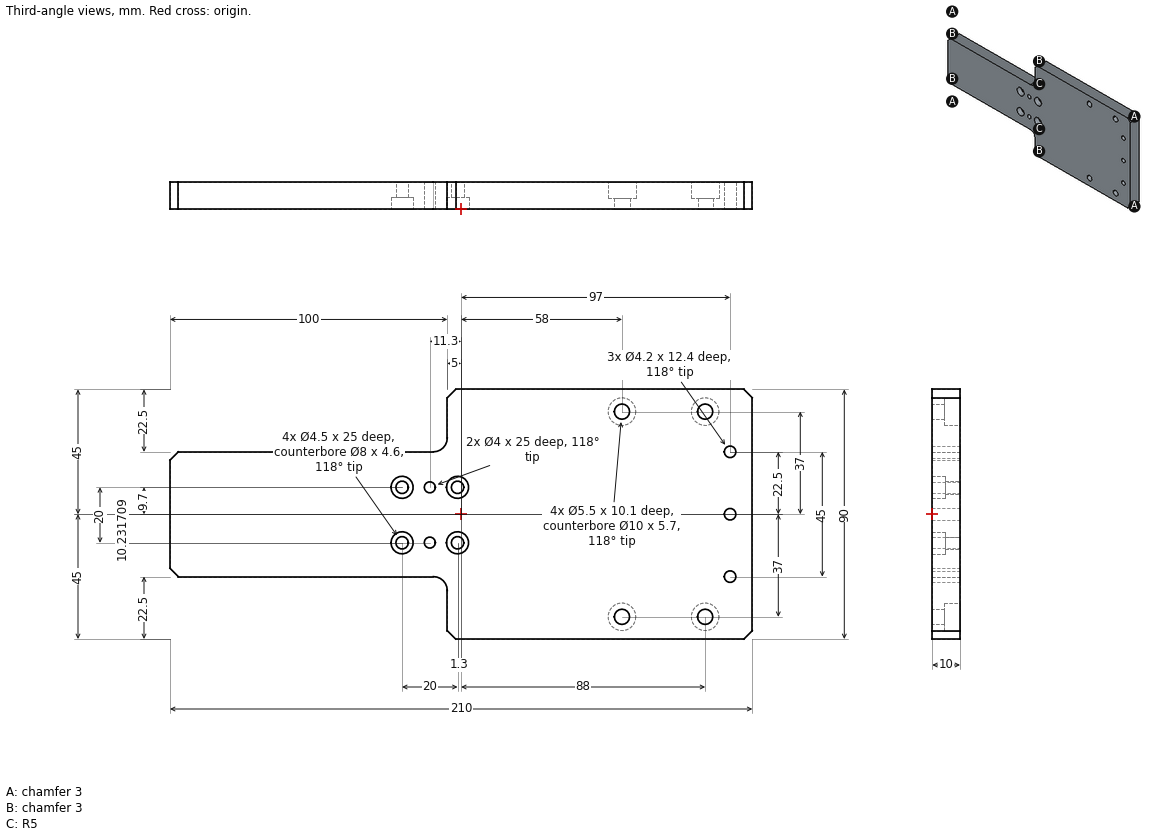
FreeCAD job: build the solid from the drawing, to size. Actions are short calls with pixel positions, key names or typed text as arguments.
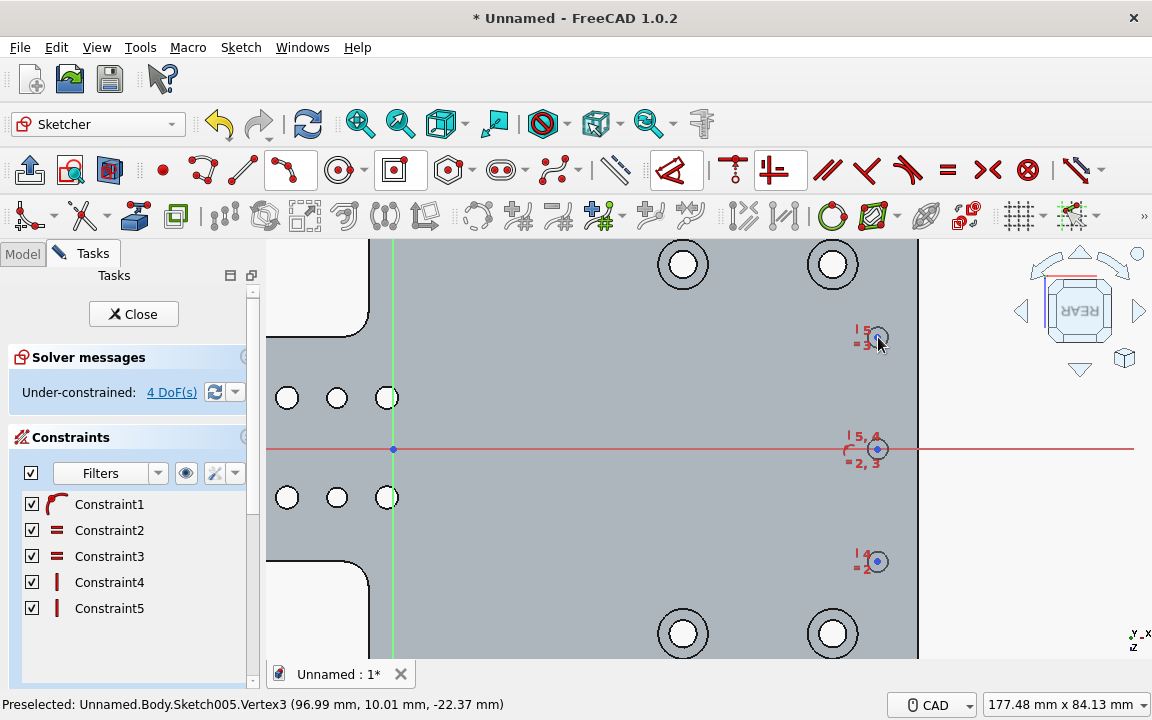
scroll(885, 555, up, 4)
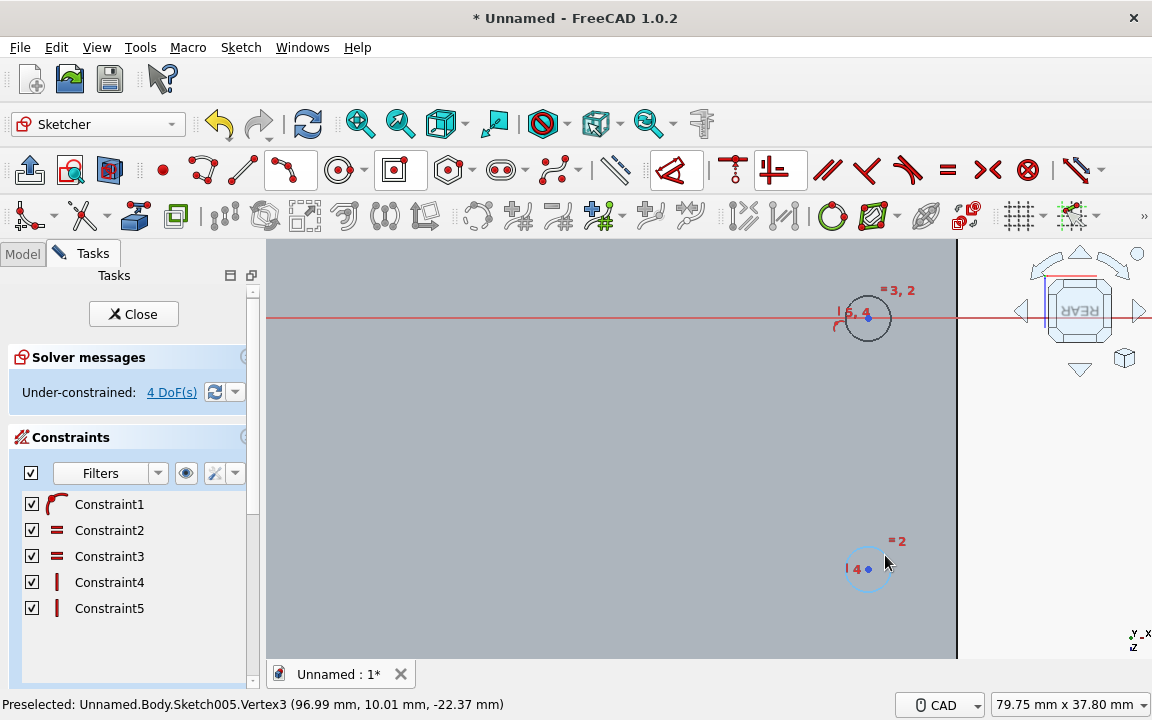
click(884, 553)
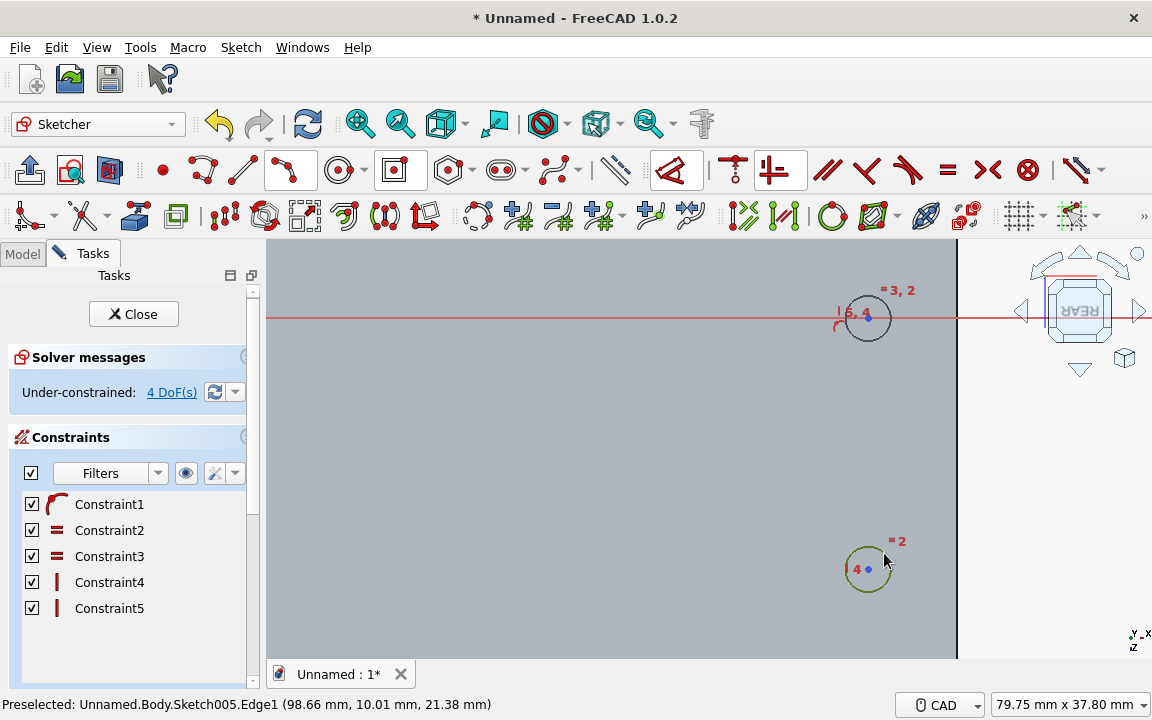
key(k)
key(o)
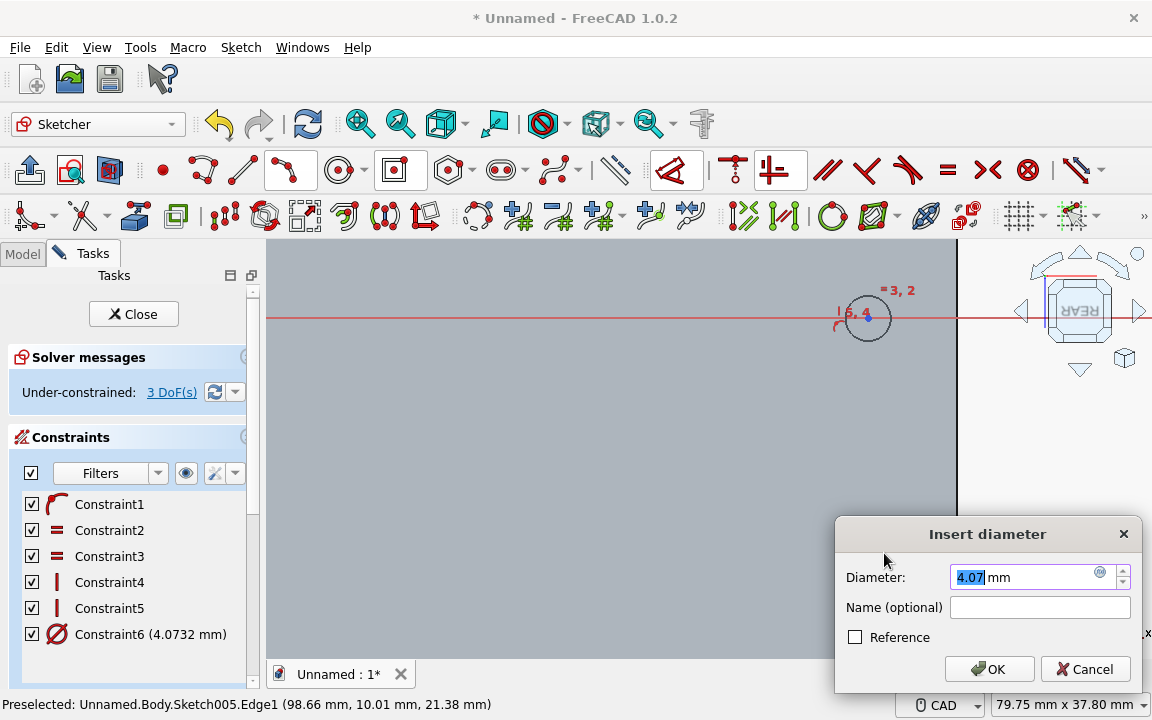
text(4.2)
key(Return)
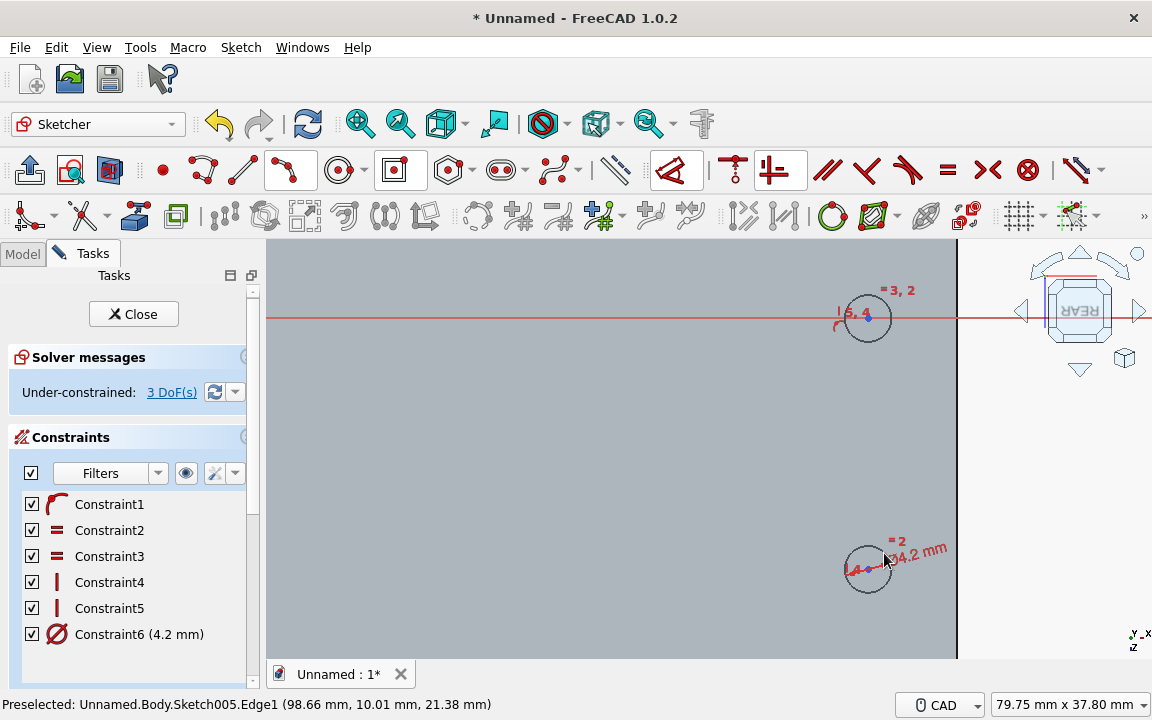
click(868, 569)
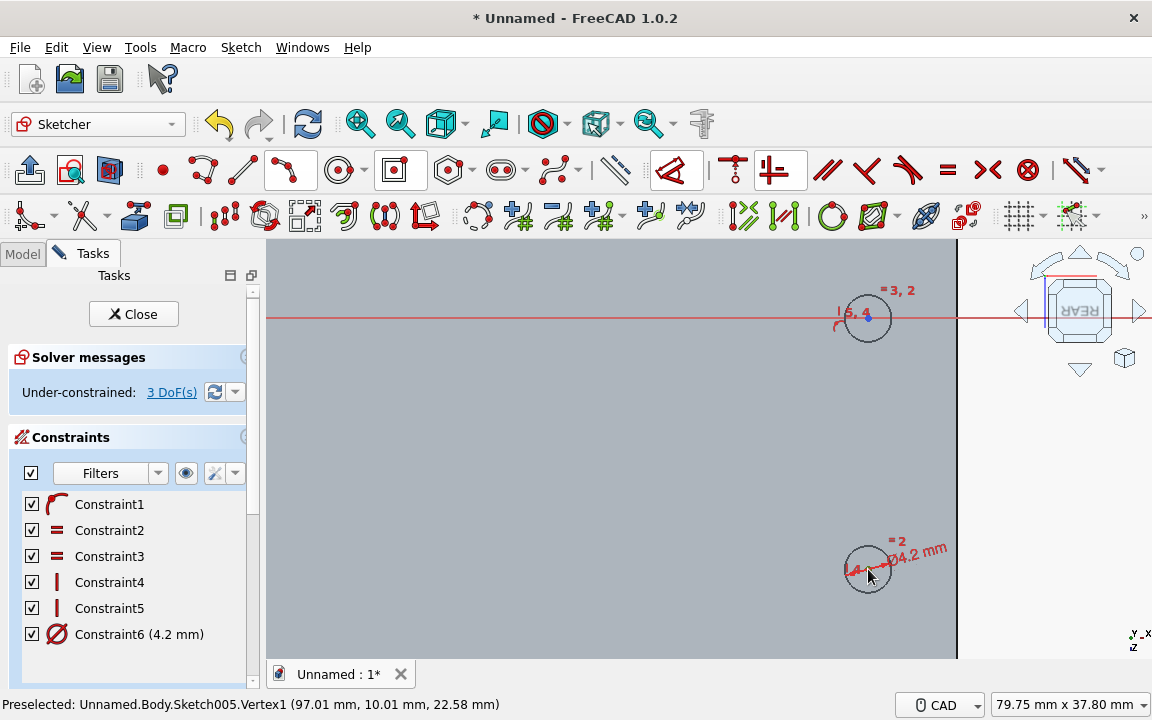
key(l)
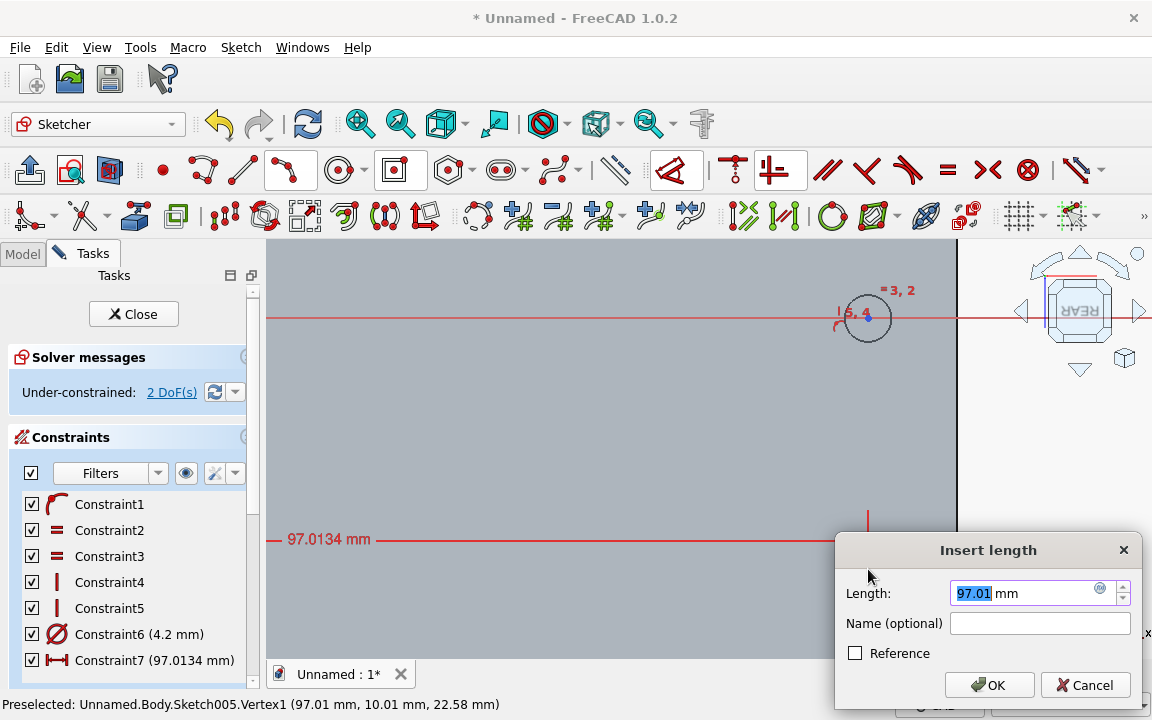
text(97)
key(Return)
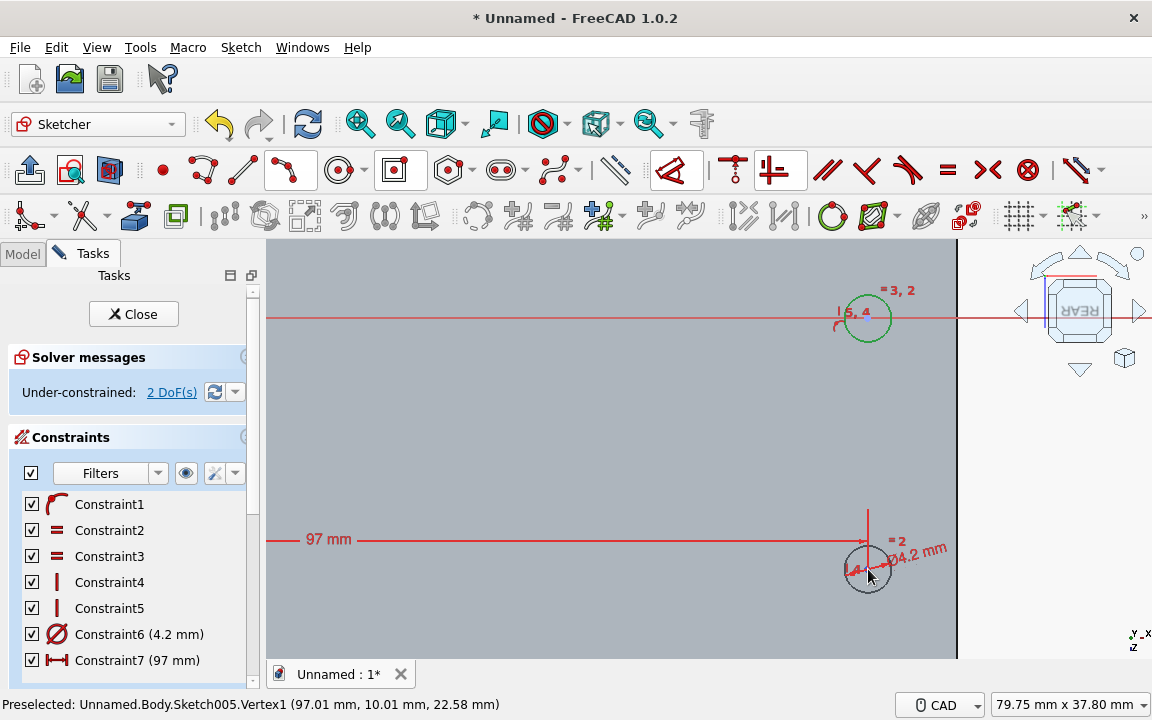
click(868, 569)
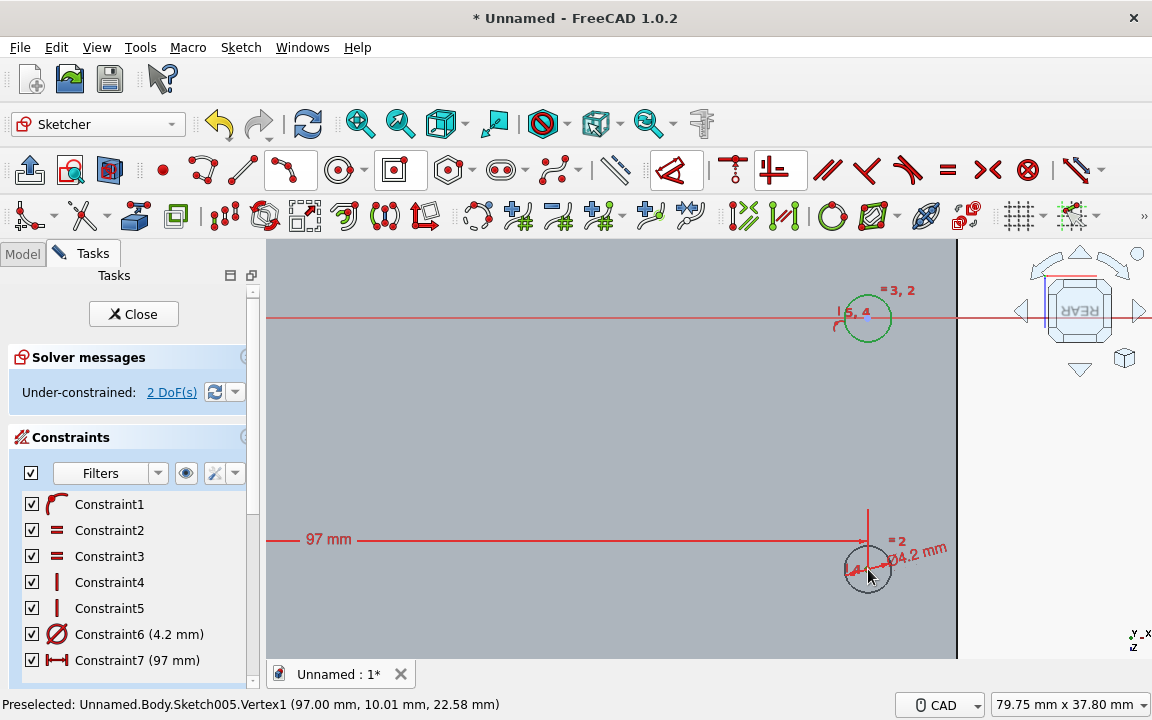
scroll(885, 555, down, 4)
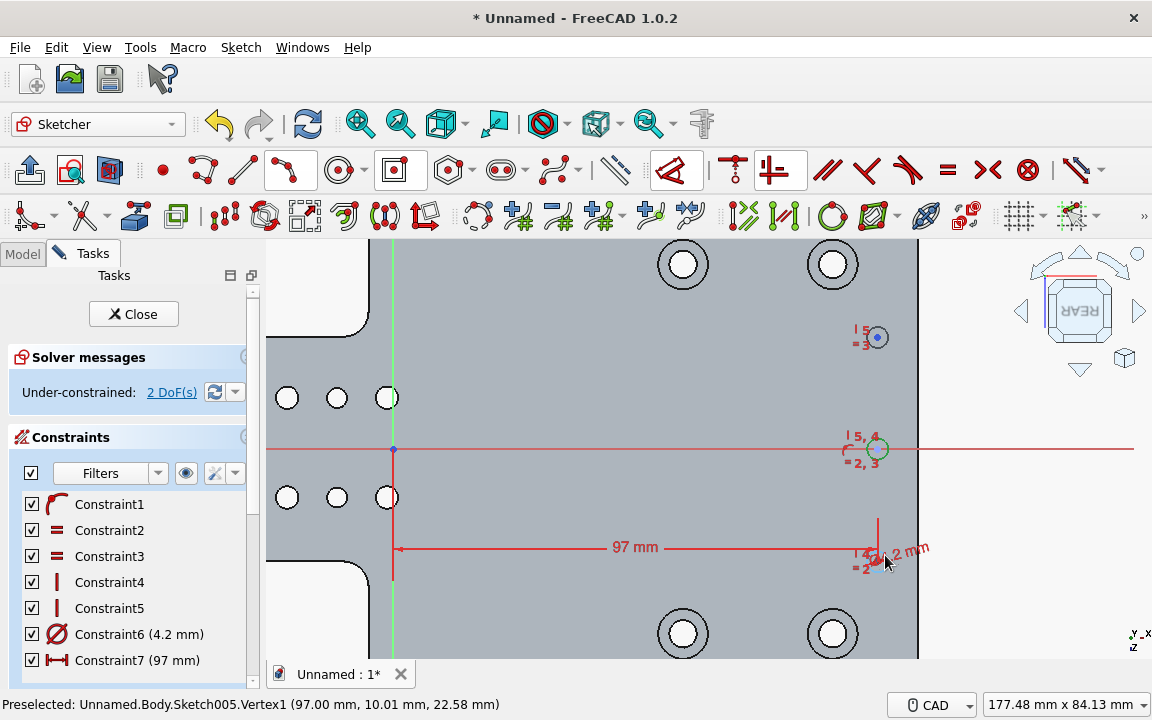
click(878, 337)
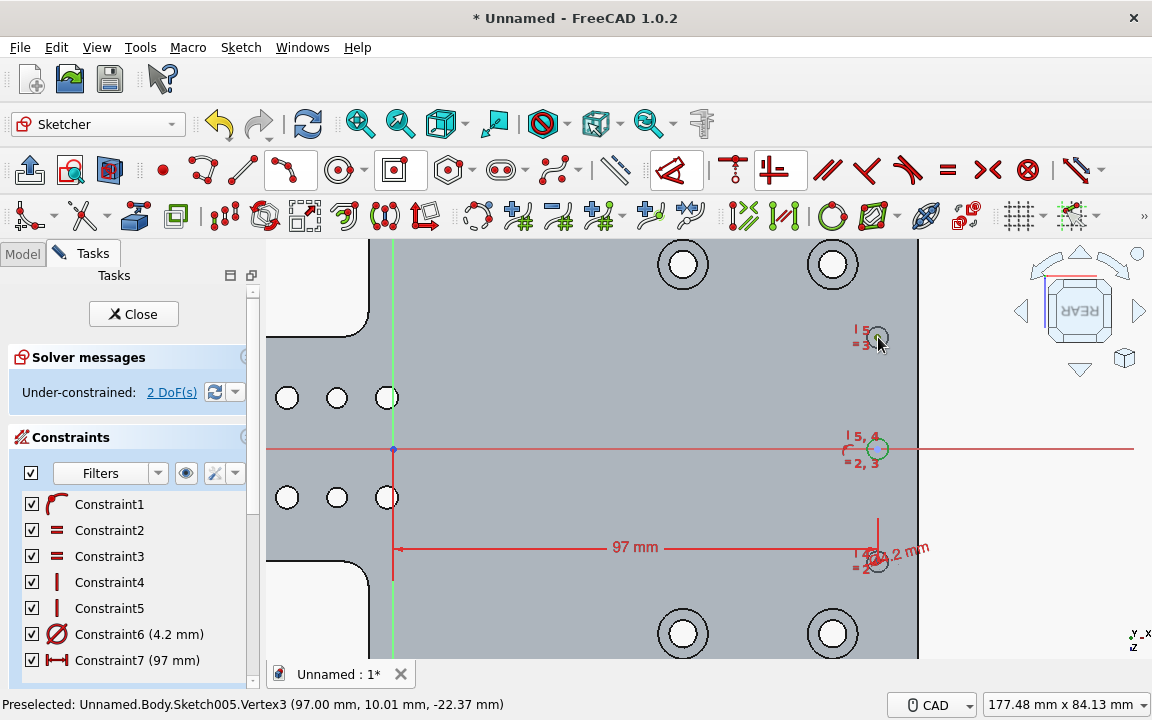
key(i)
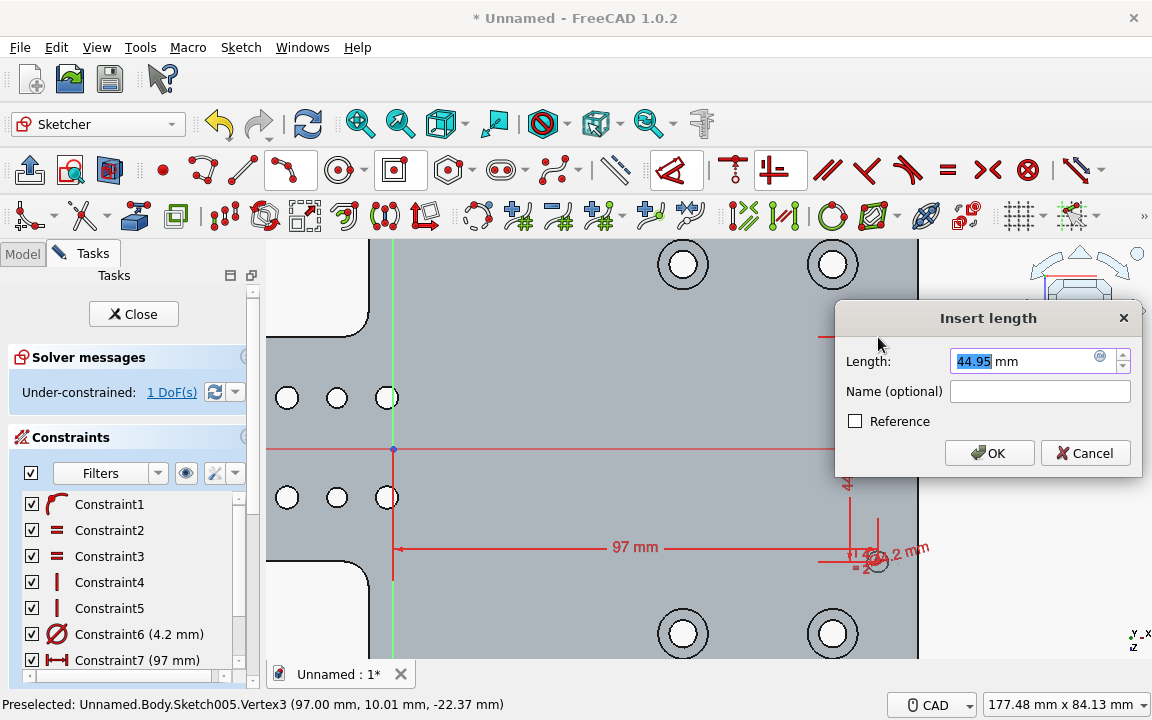
text(45)
key(Return)